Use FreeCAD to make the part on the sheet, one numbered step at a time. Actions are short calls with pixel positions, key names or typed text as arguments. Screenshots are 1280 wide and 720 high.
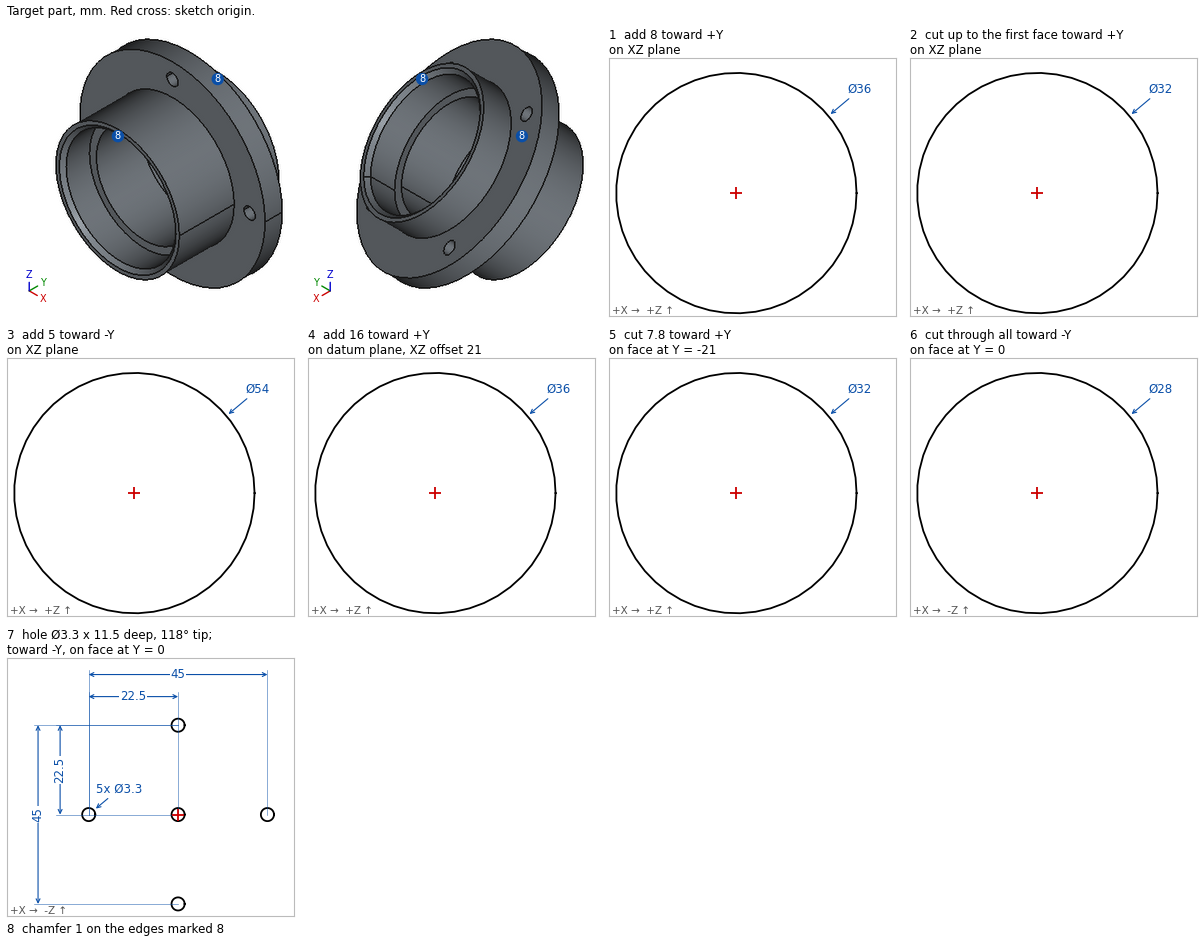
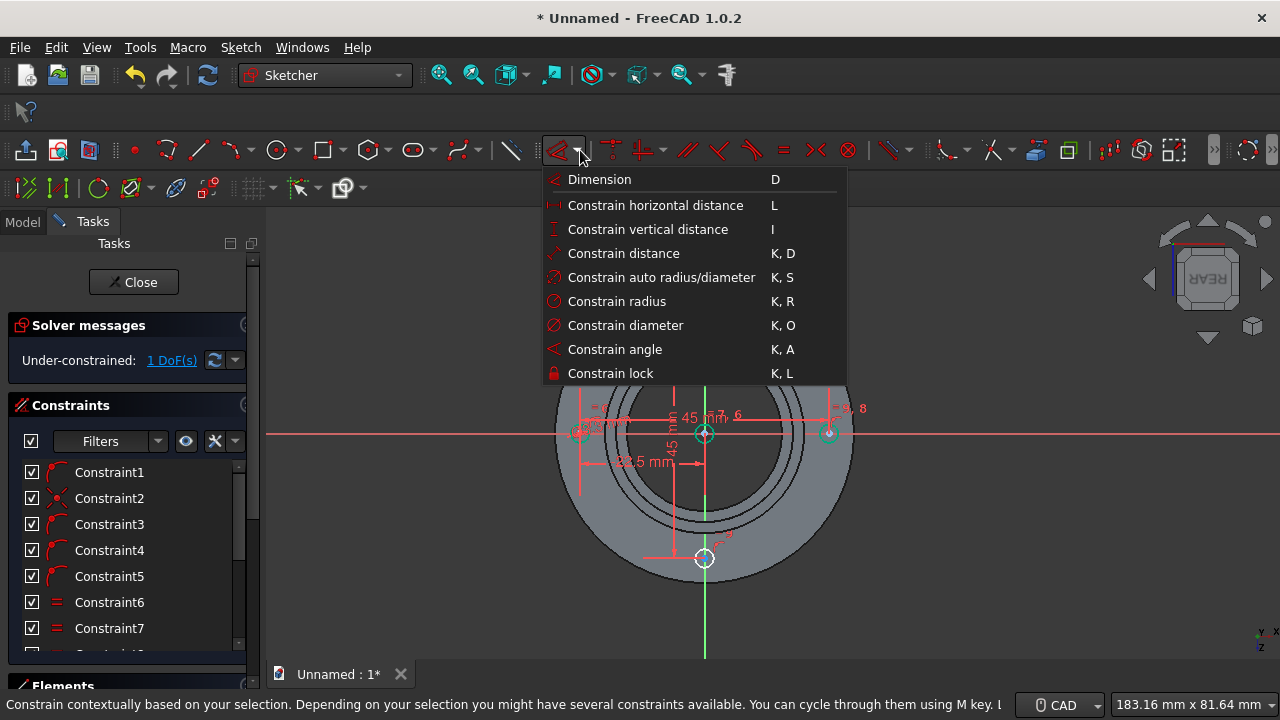
click(695, 229)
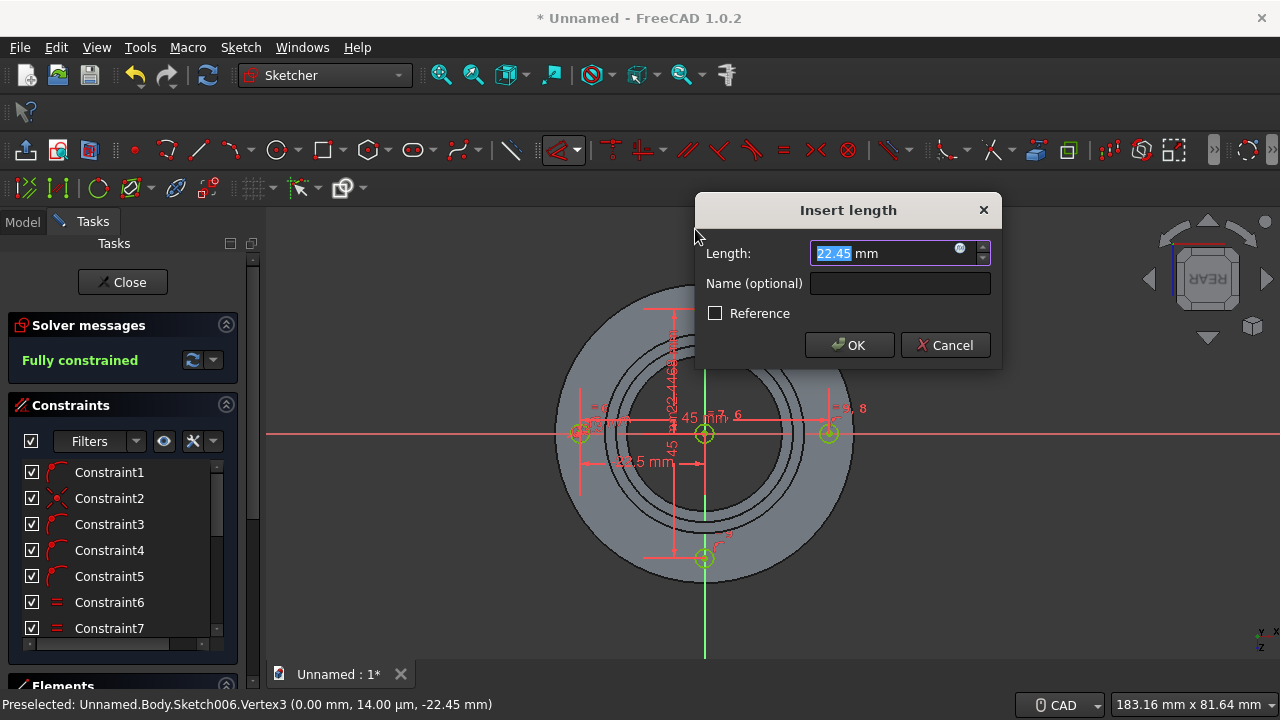
text(22.5)
key(Return)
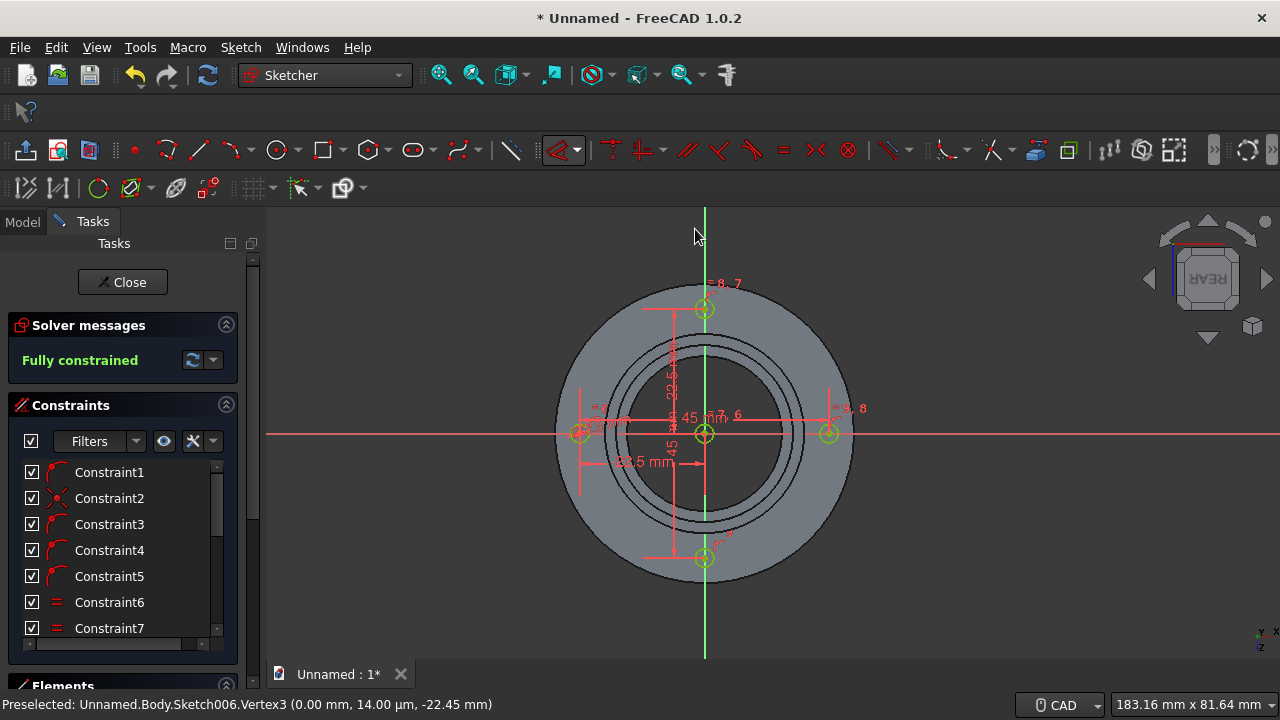
click(123, 282)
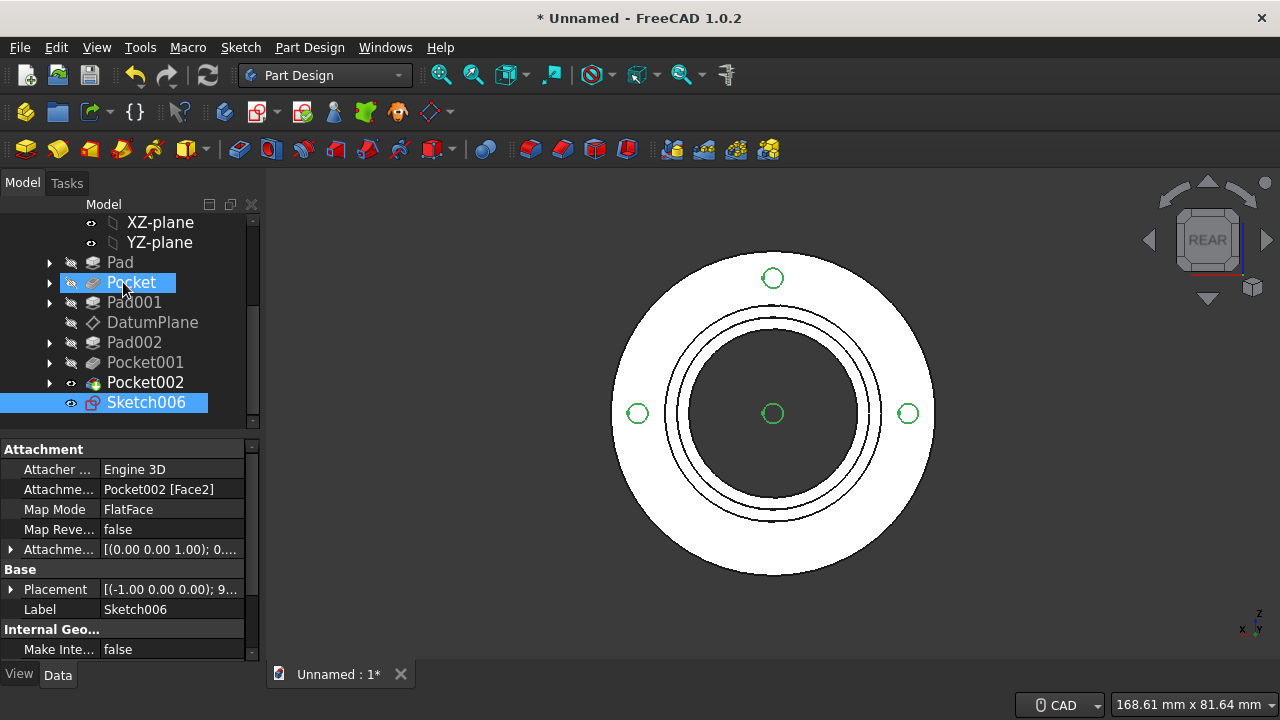
click(272, 150)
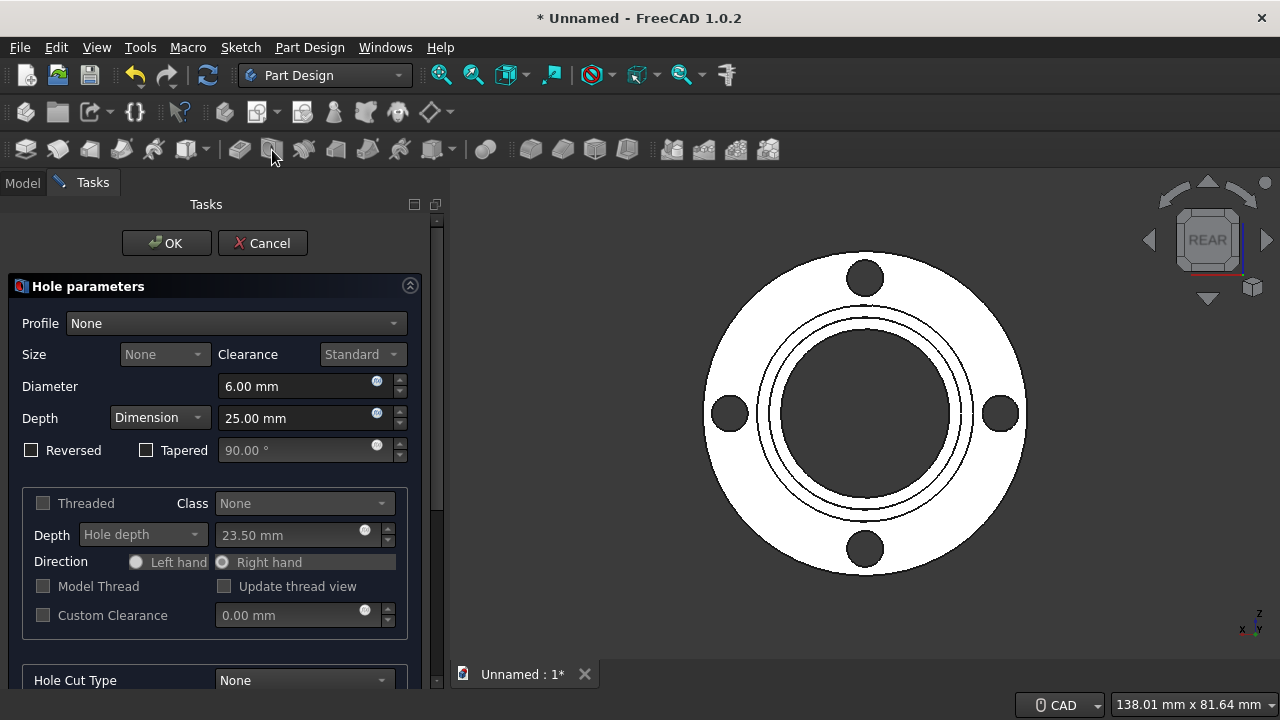
triple_click(305, 386)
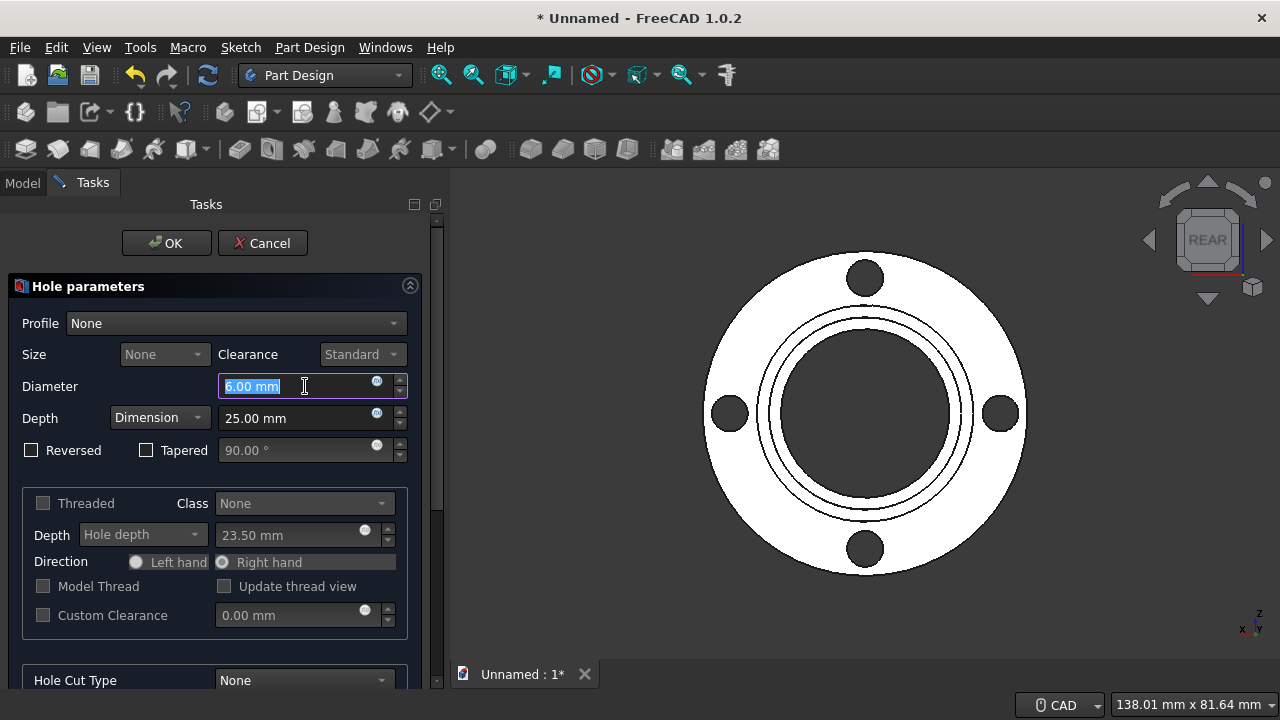
text(3.3)
key(Tab)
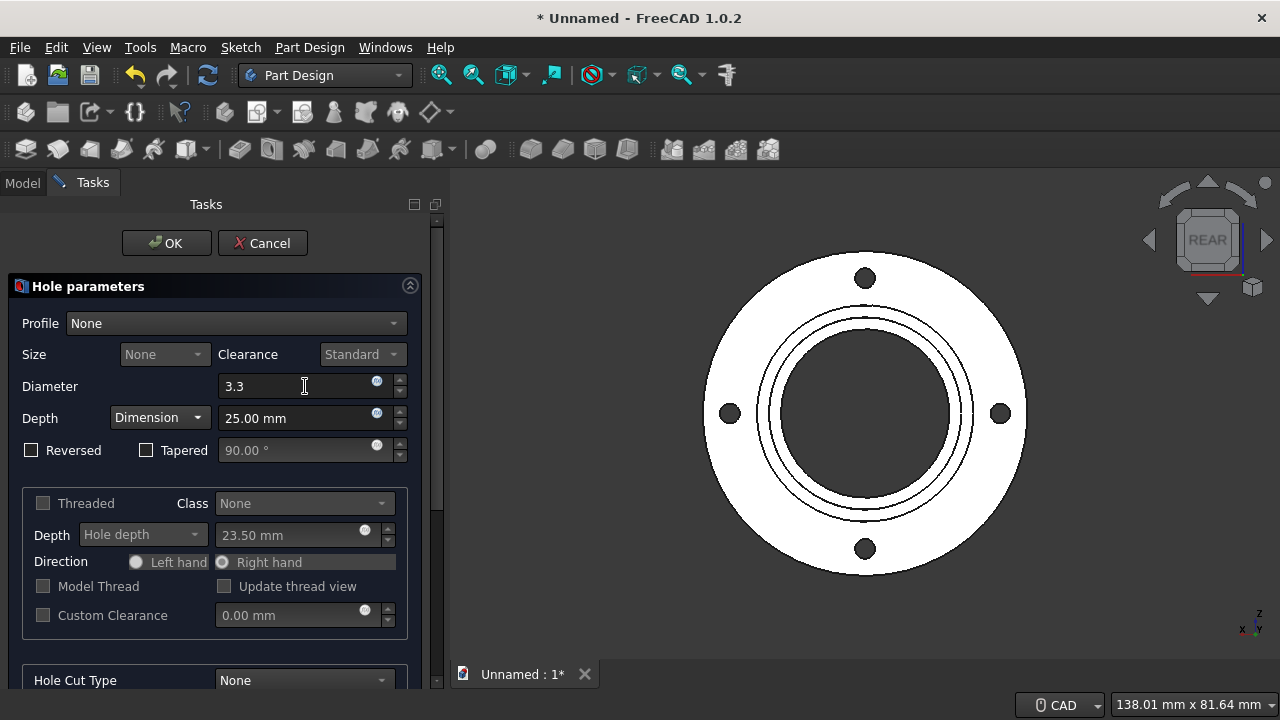
triple_click(305, 418)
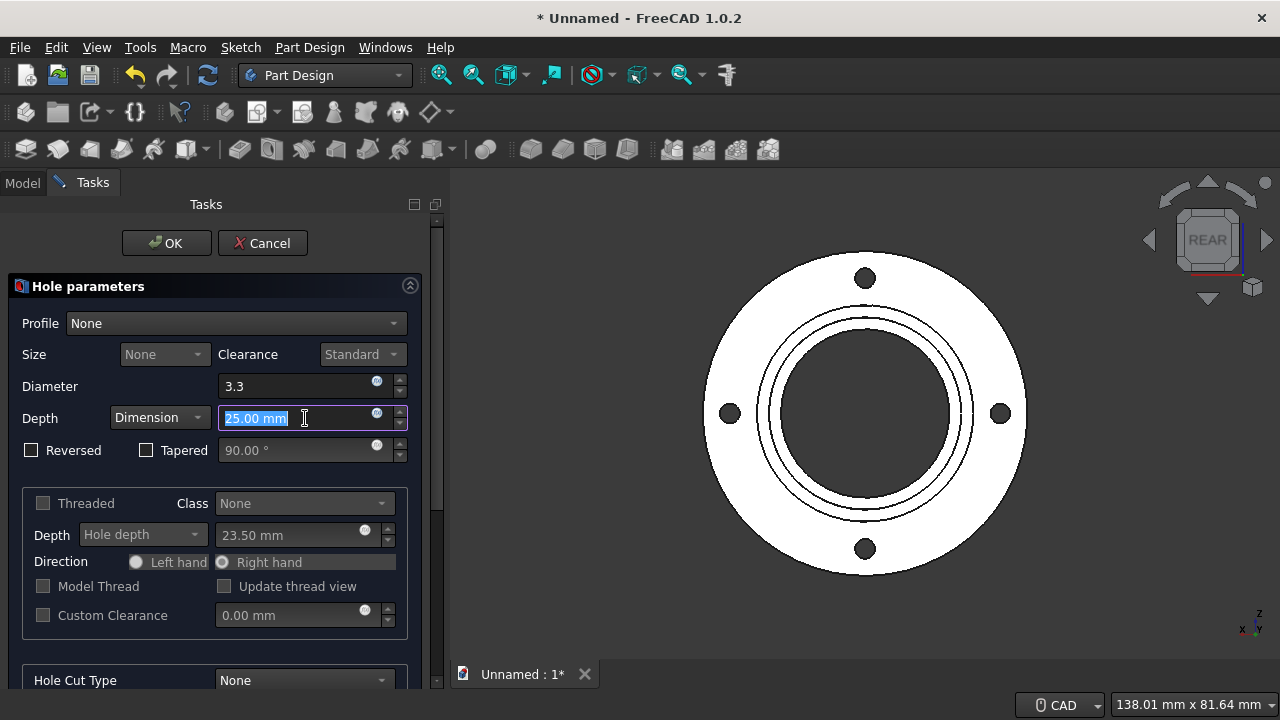
text(11.5)
key(Tab)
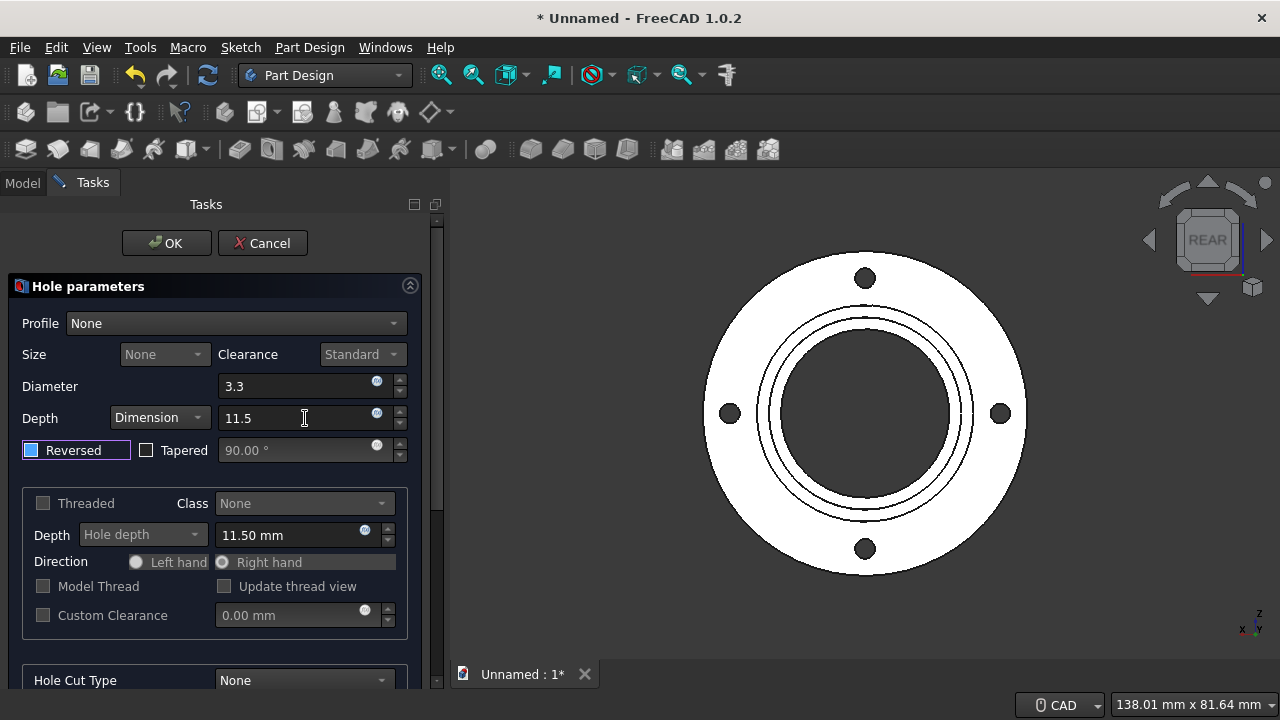
click(167, 243)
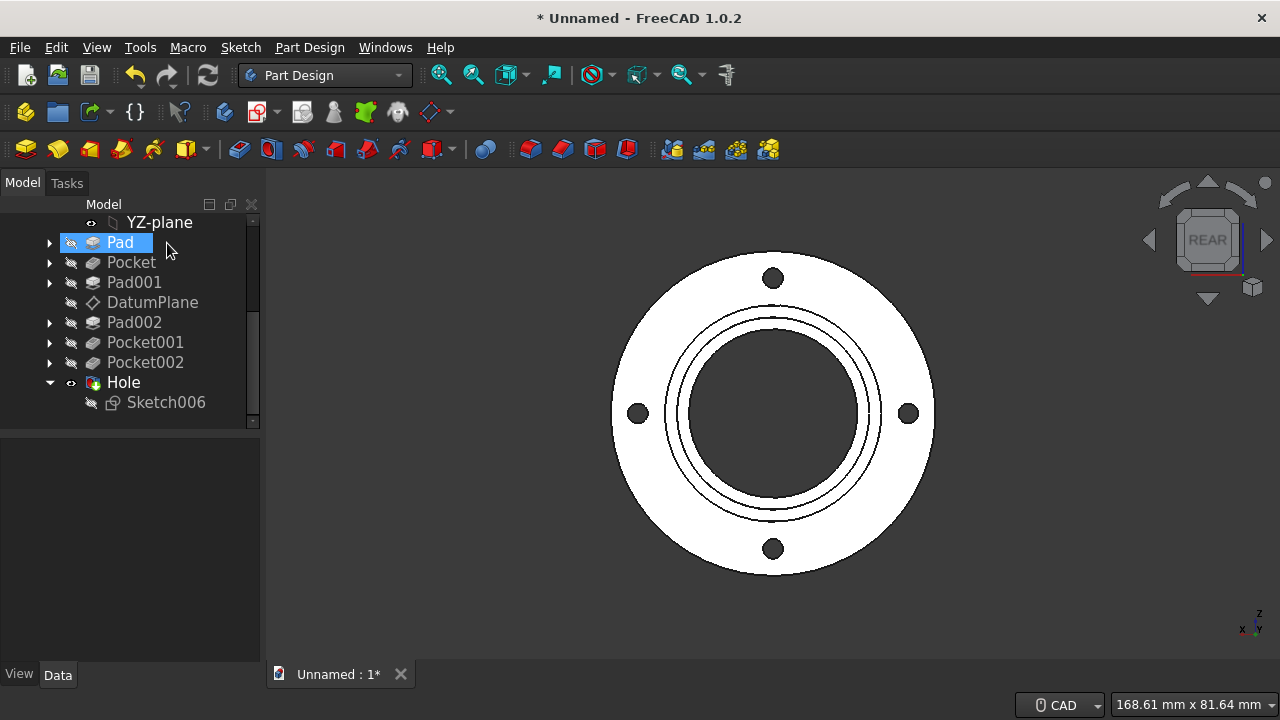
click(851, 356)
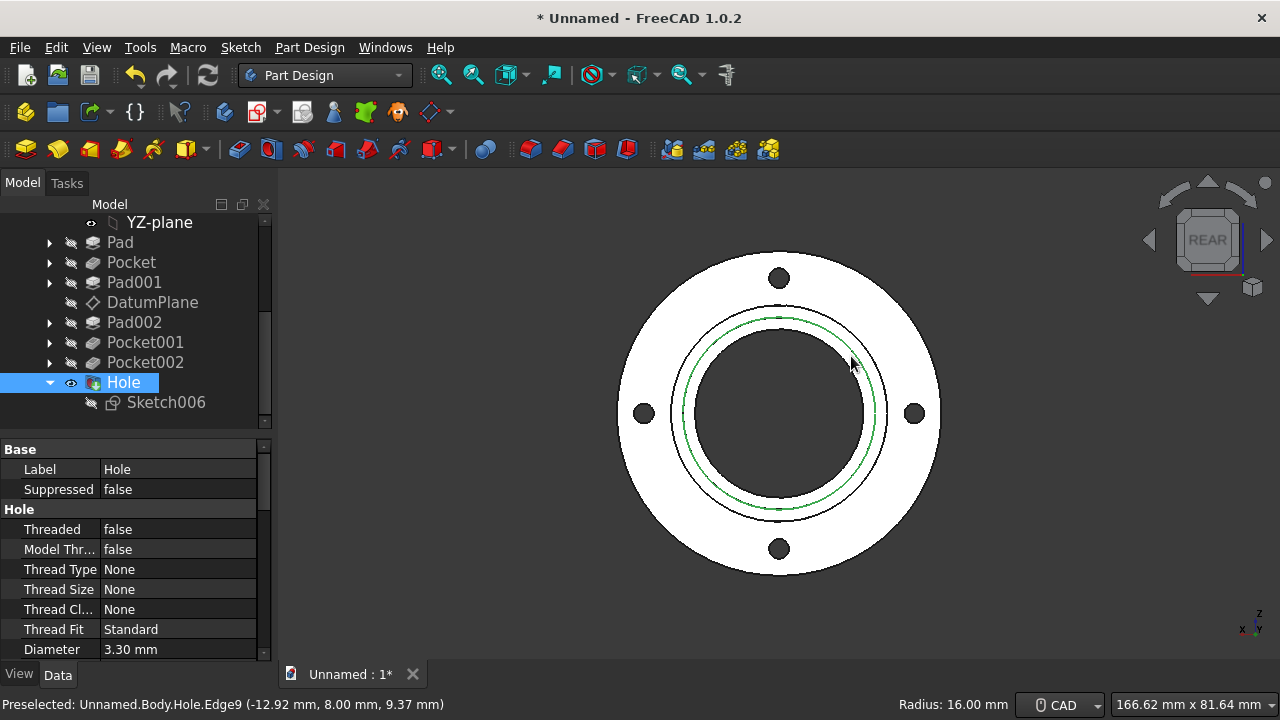
key(0)